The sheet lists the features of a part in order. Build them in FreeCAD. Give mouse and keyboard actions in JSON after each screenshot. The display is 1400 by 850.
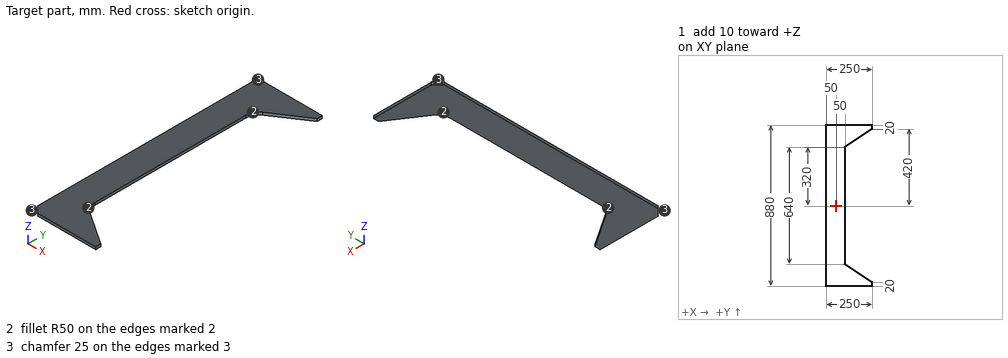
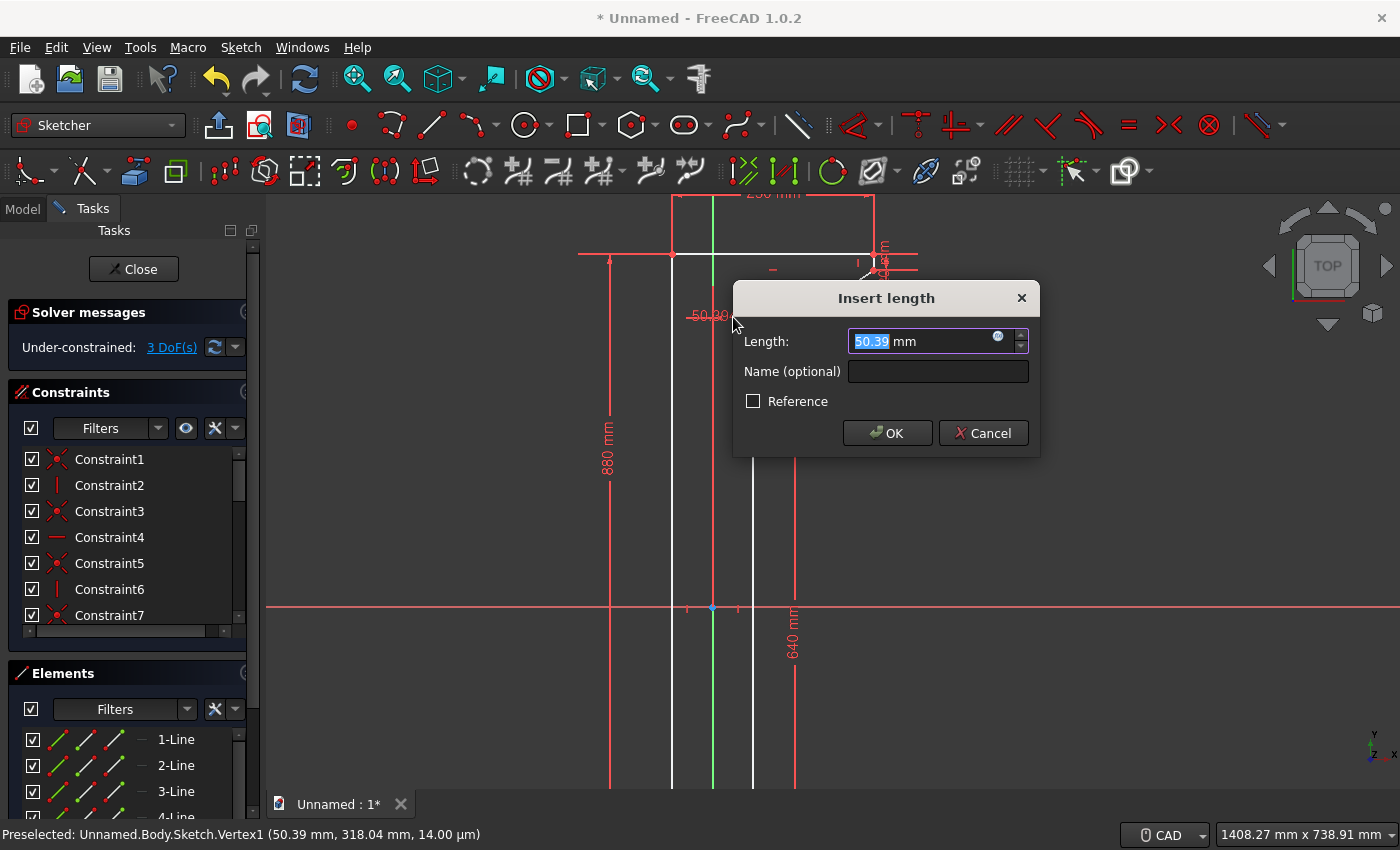
{"action": "type", "text": "50"}
{"action": "key", "text": "Return"}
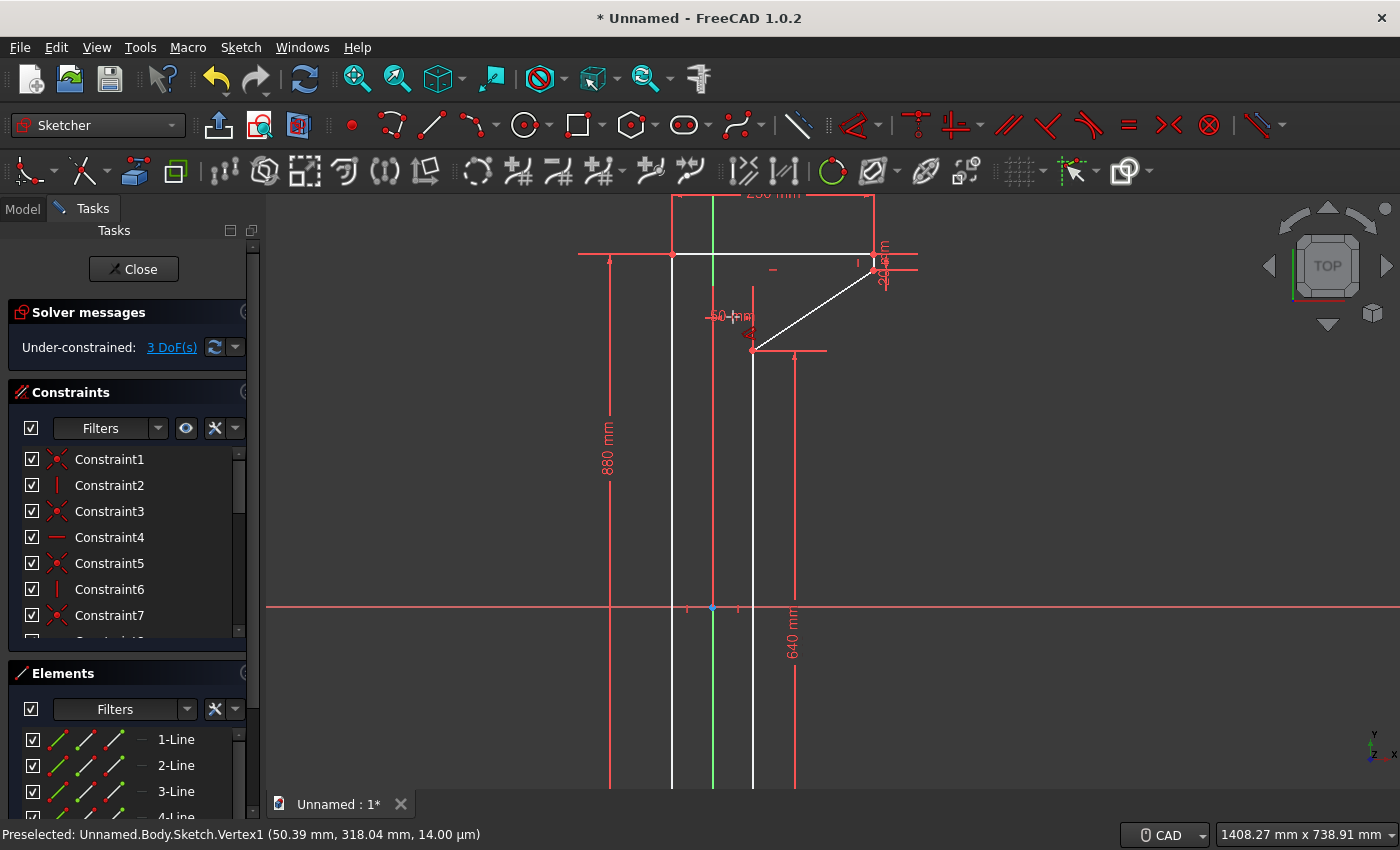
{"action": "left_click", "coordinate": [672, 254]}
{"action": "left_click", "coordinate": [693, 641]}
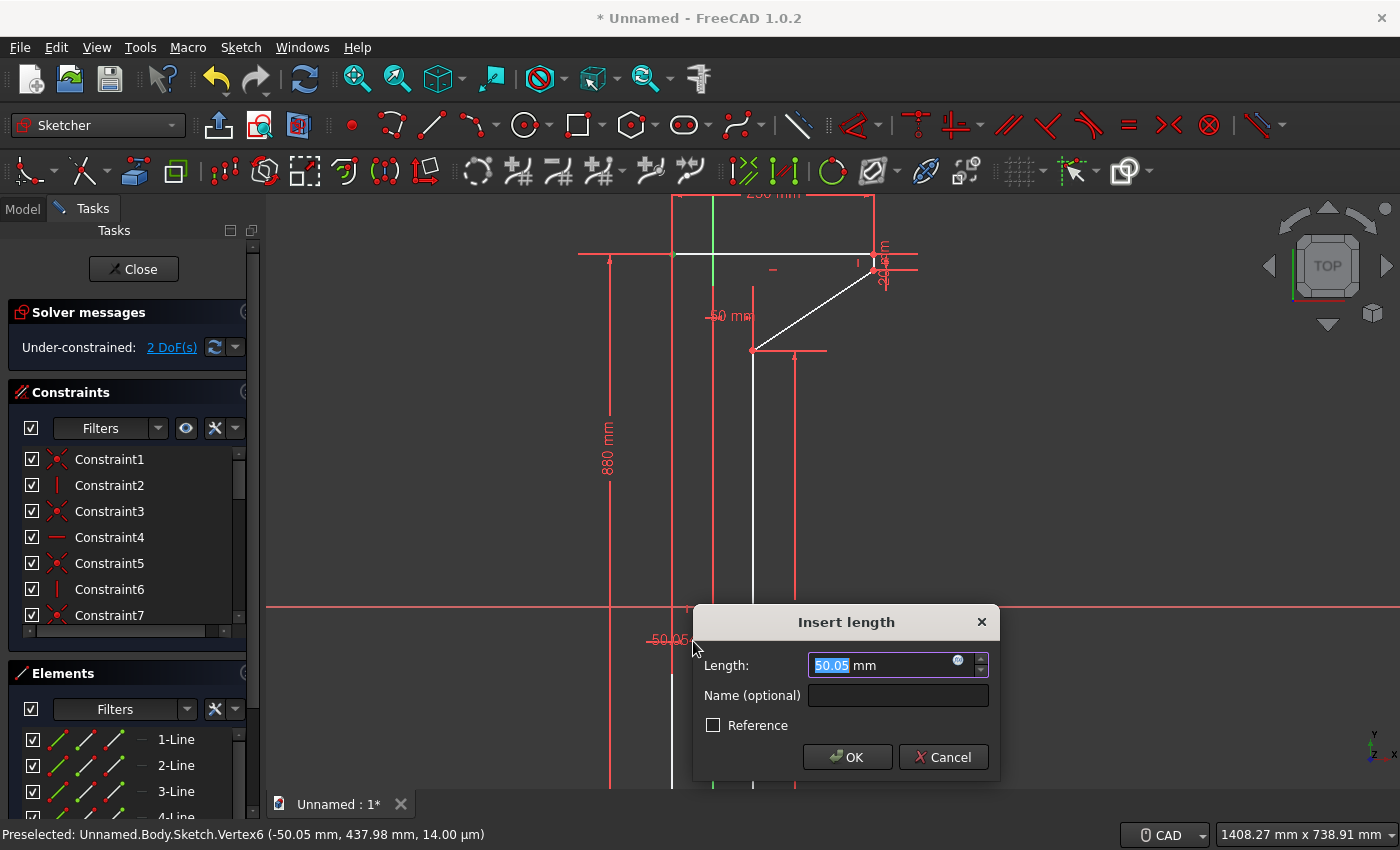
{"action": "type", "text": "50"}
{"action": "key", "text": "Return"}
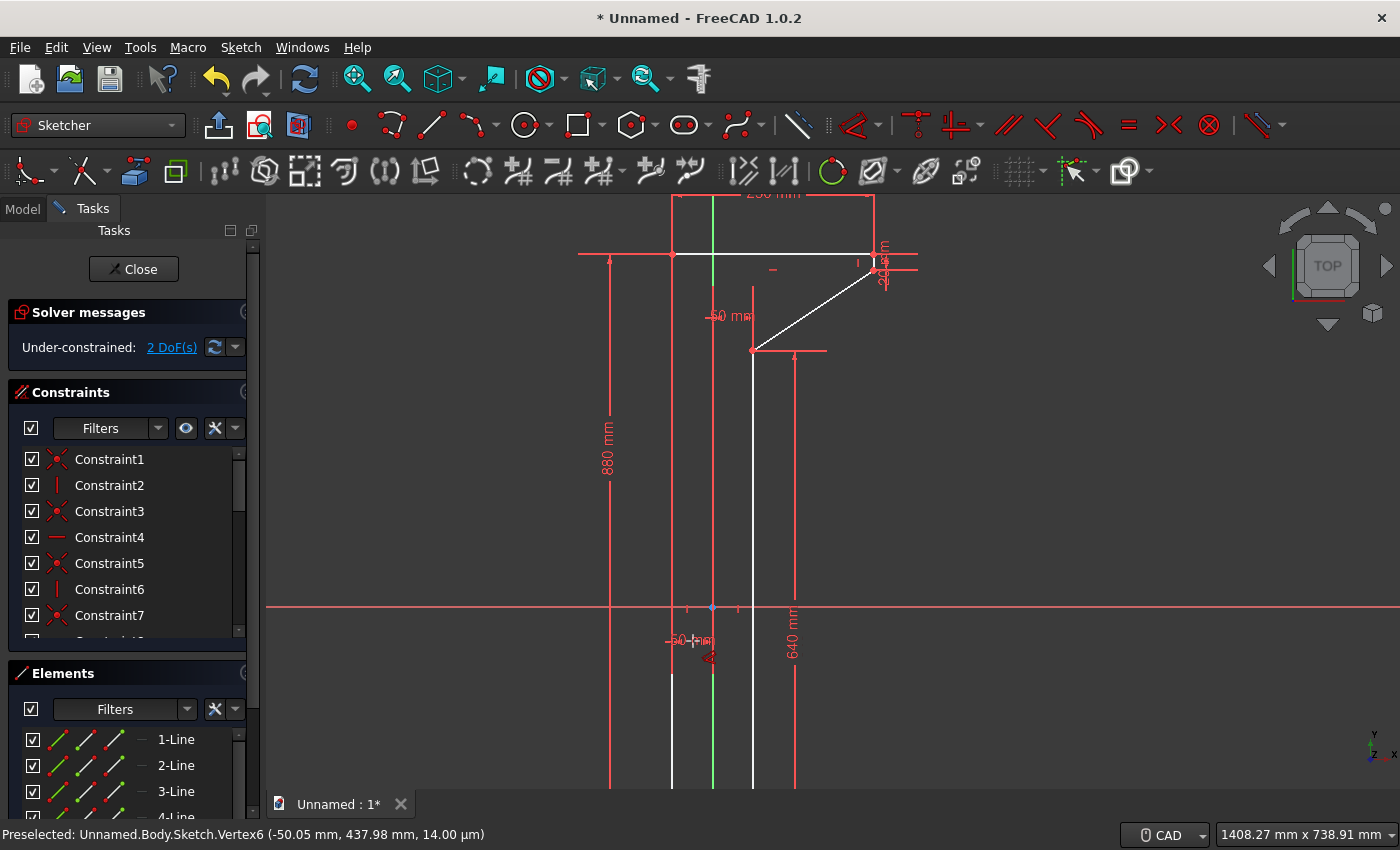
{"action": "left_click", "coordinate": [753, 351]}
{"action": "left_click", "coordinate": [787, 479]}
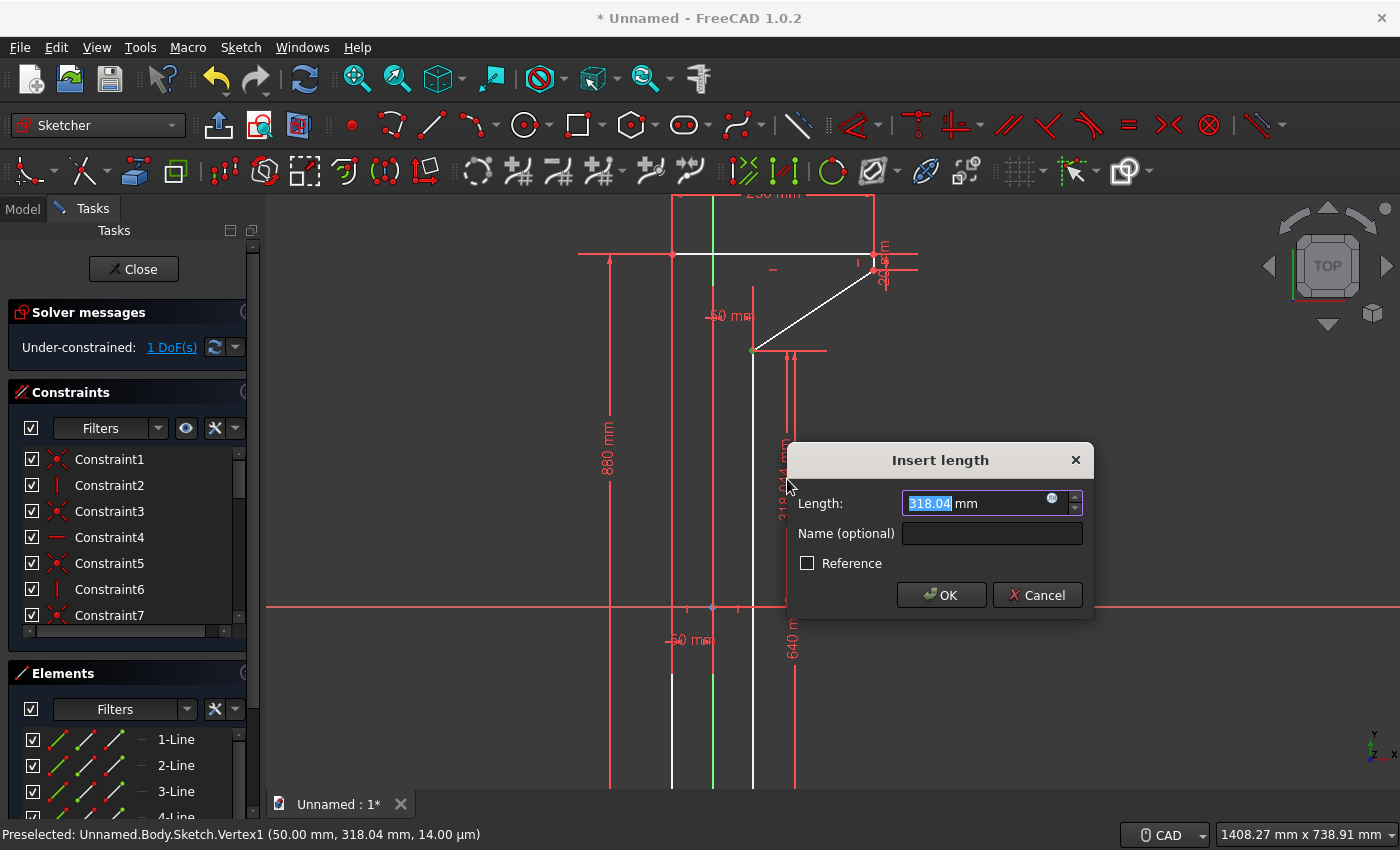
{"action": "type", "text": "320"}
{"action": "key", "text": "Return"}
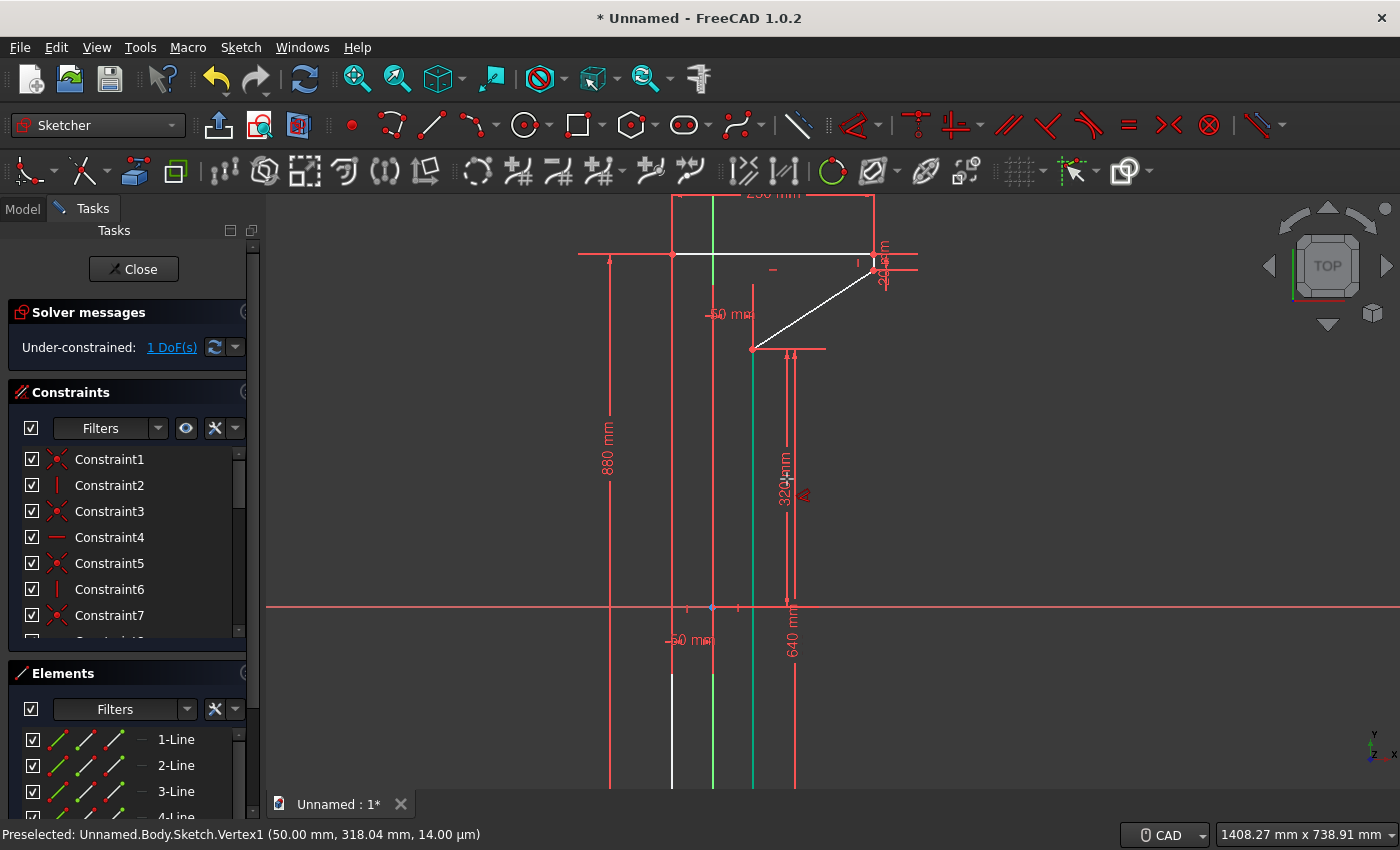
{"action": "left_click", "coordinate": [874, 270]}
{"action": "left_click", "coordinate": [908, 439]}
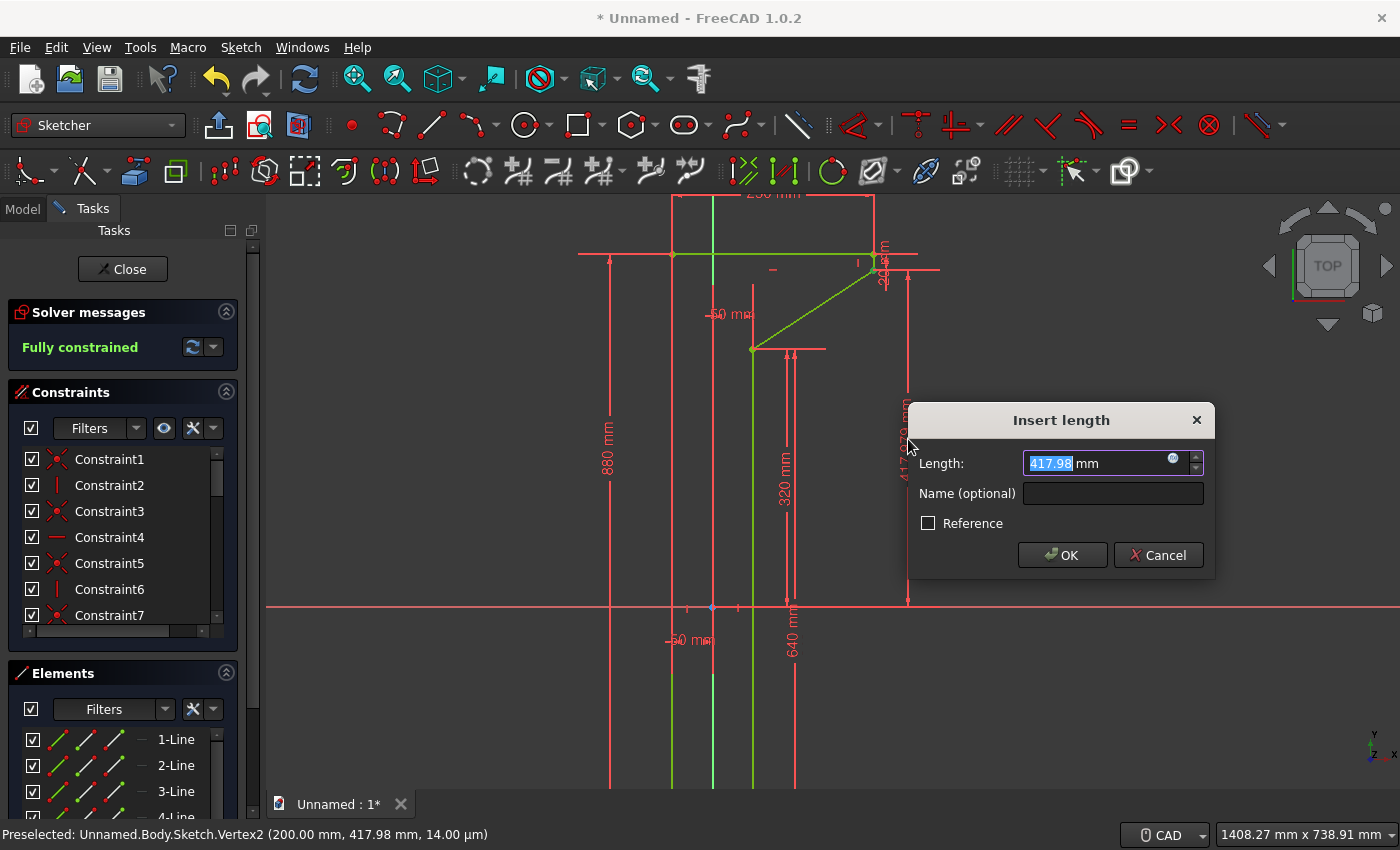
{"action": "type", "text": "420"}
{"action": "key", "text": "Return"}
{"action": "key", "text": "Escape"}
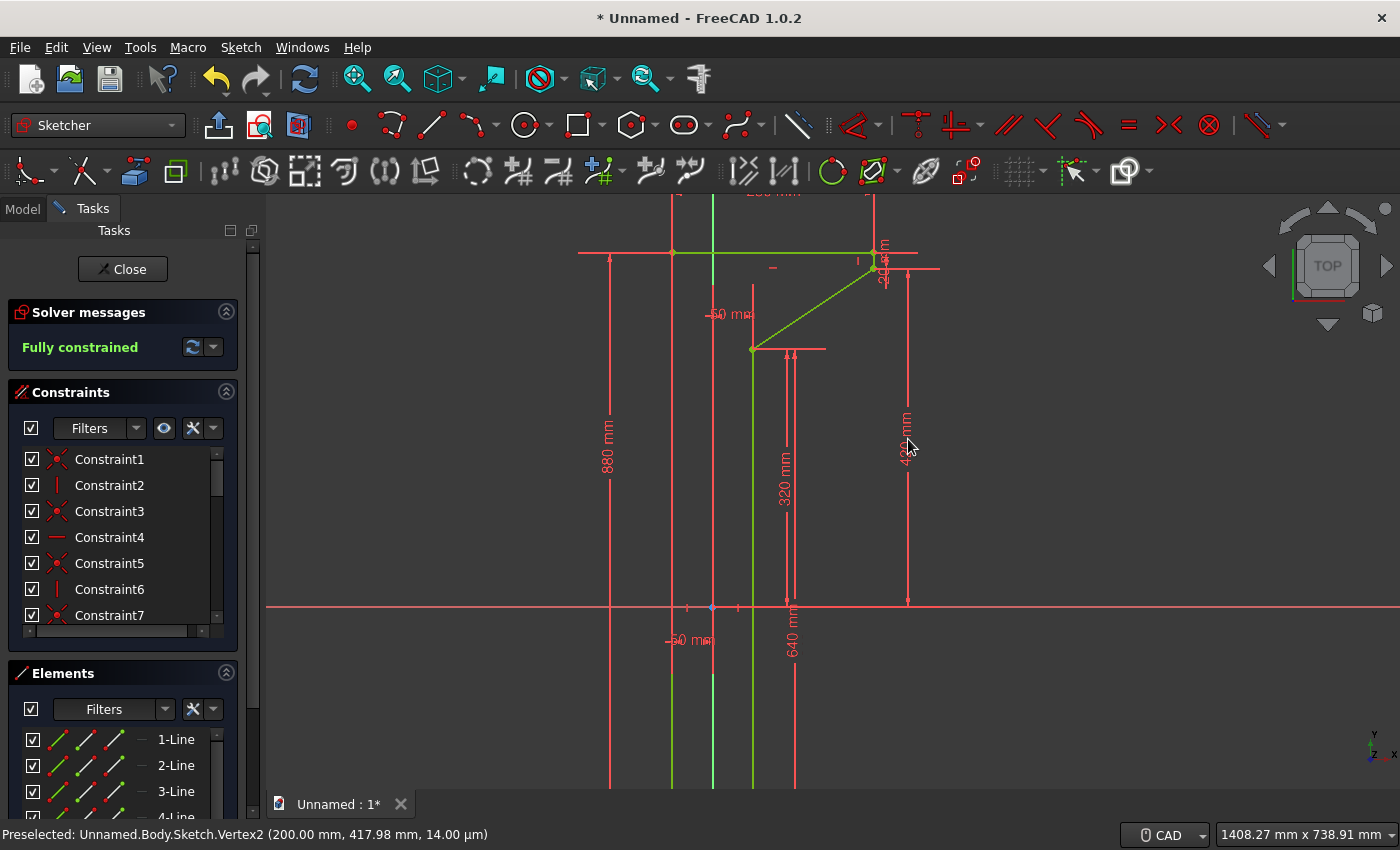
{"action": "left_click", "coordinate": [123, 269]}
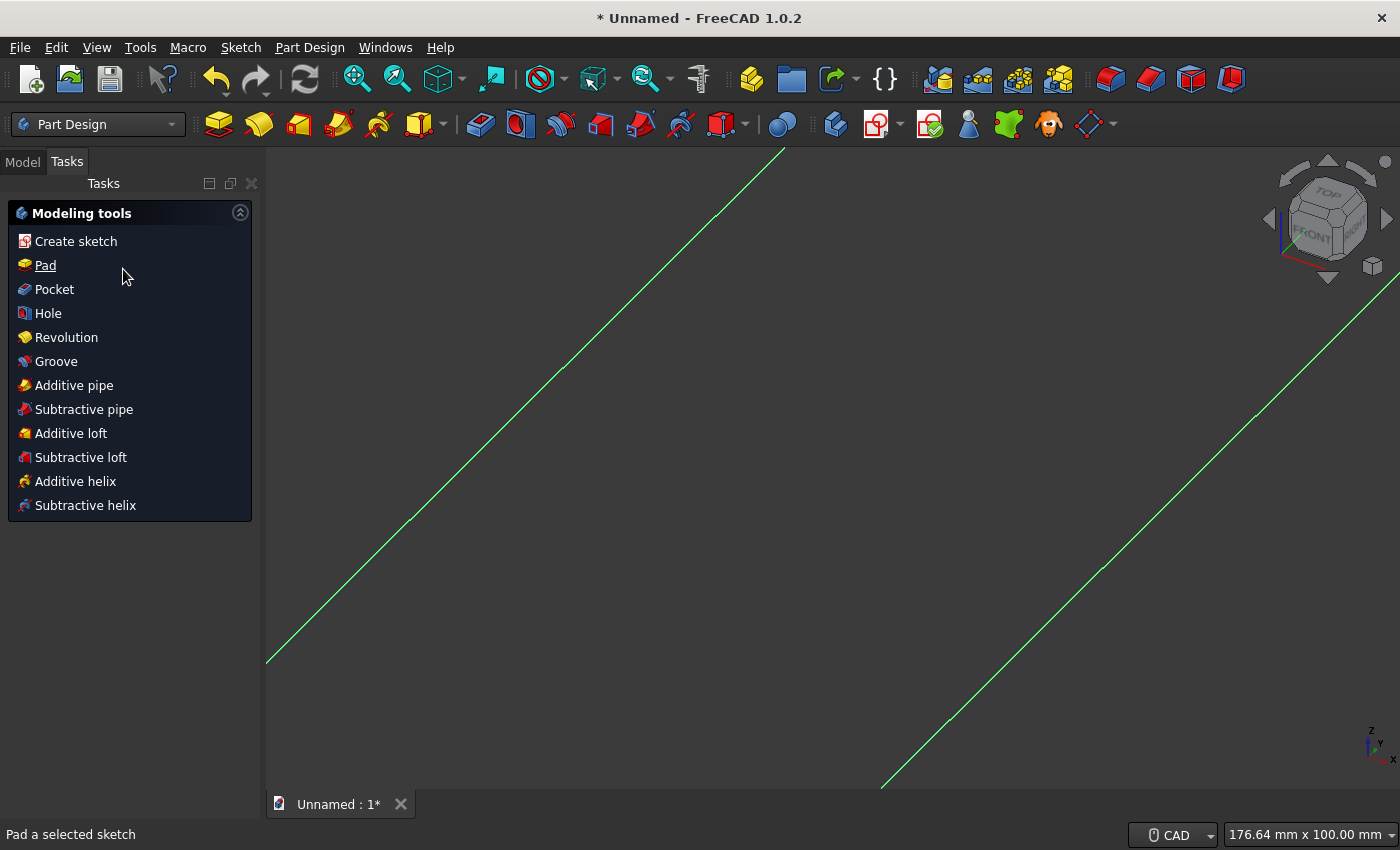
{"action": "left_click", "coordinate": [220, 124]}